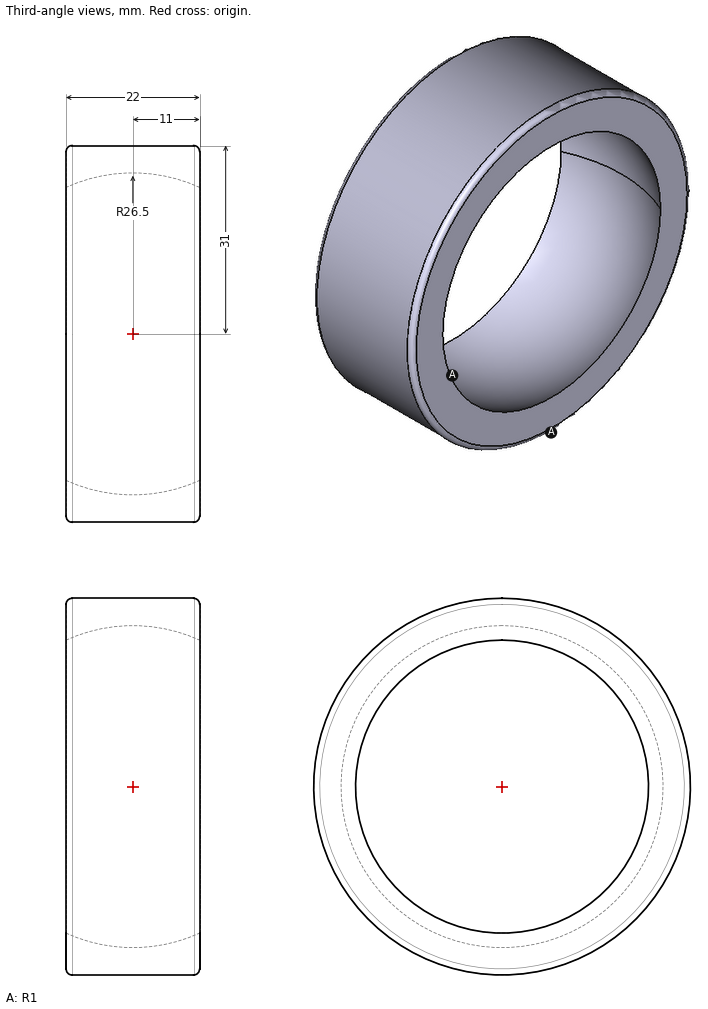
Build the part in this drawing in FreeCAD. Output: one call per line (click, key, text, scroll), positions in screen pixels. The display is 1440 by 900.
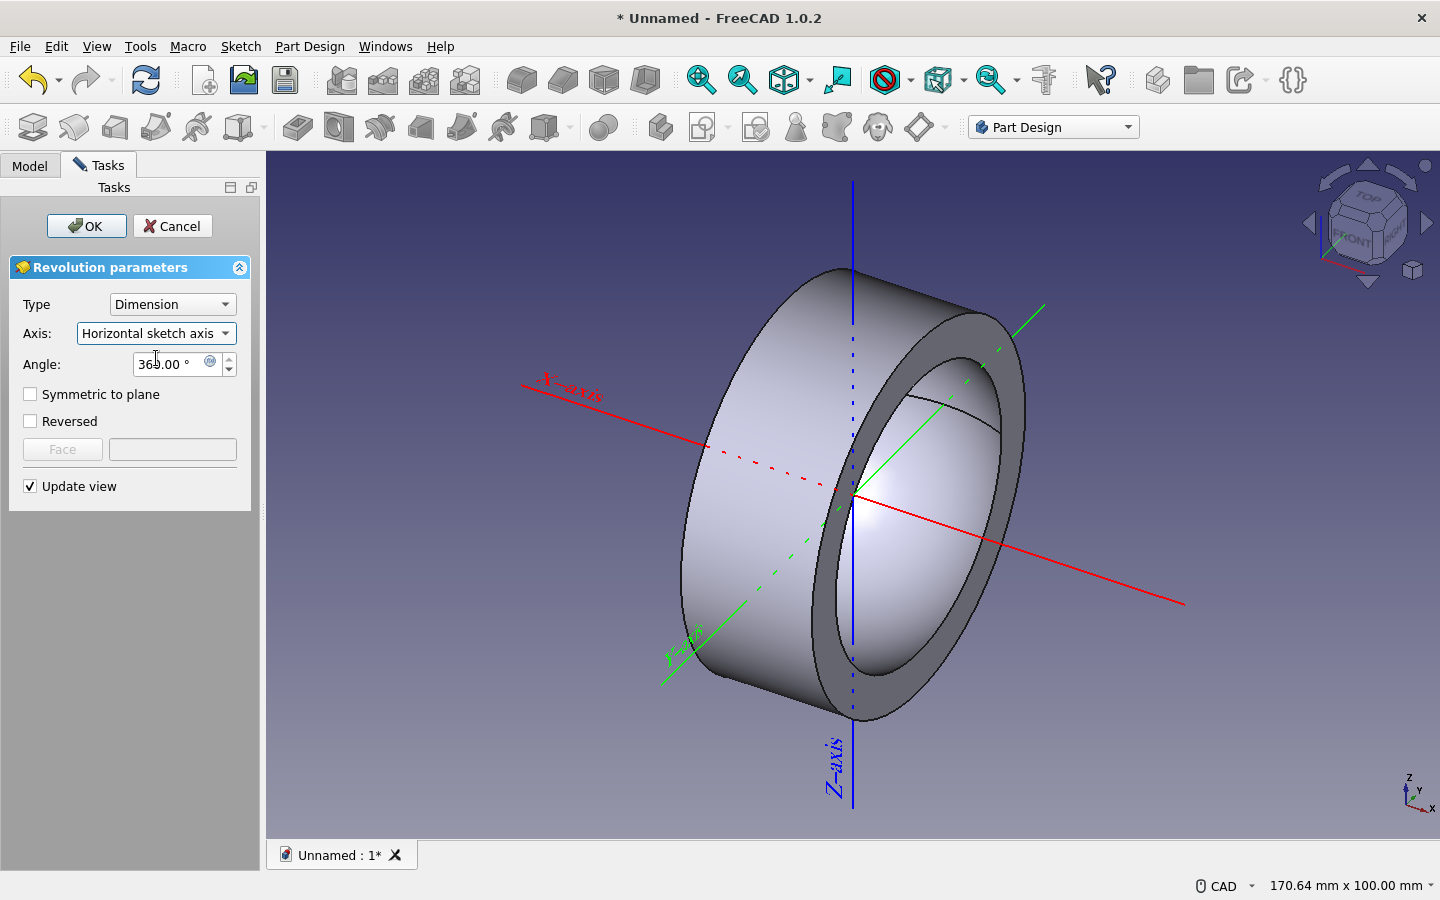
click(87, 226)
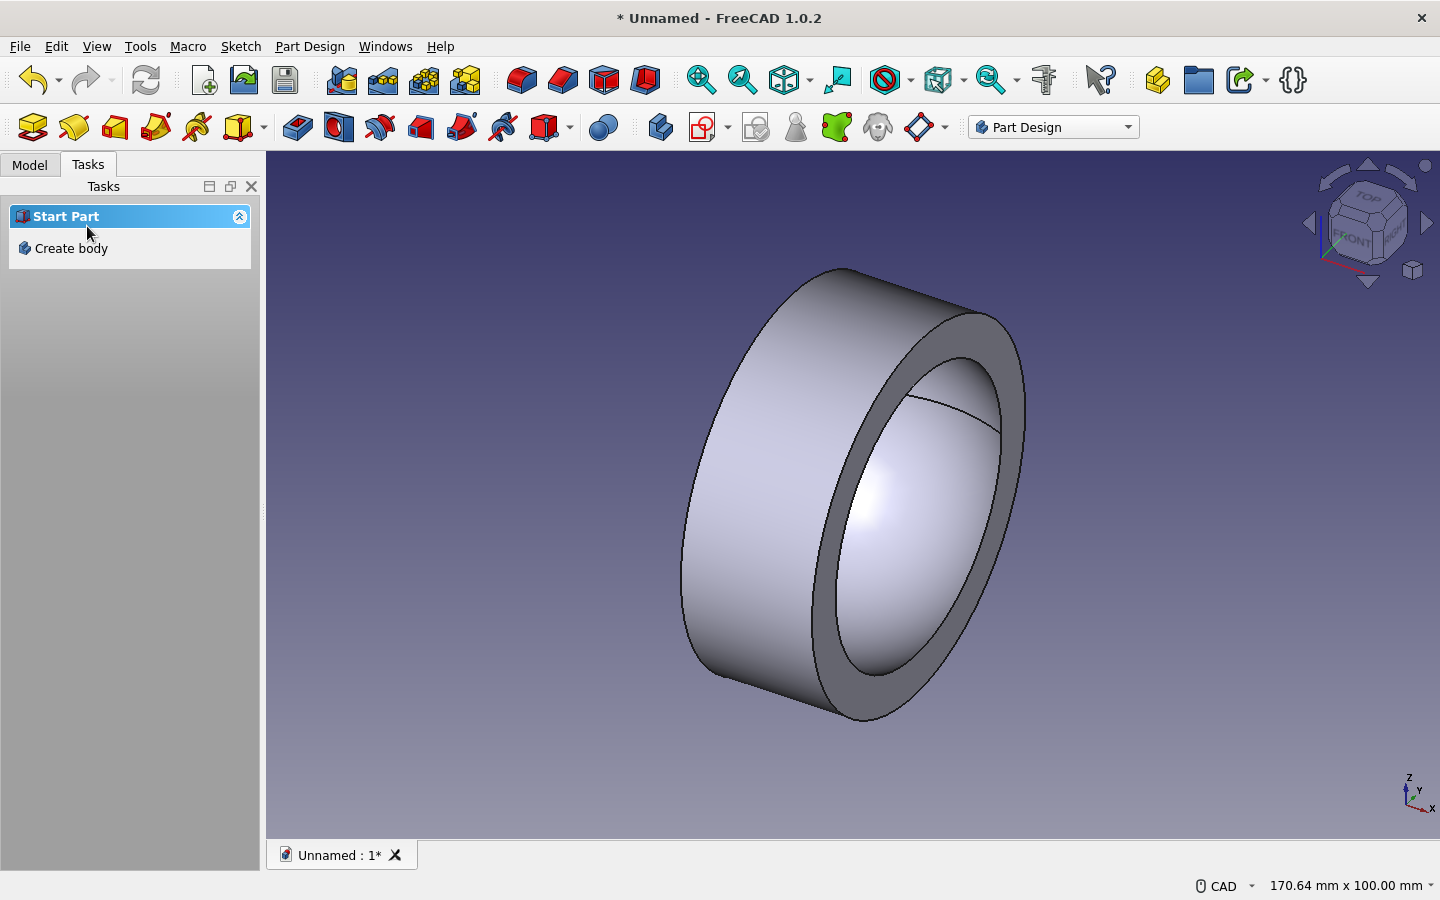
click(812, 622)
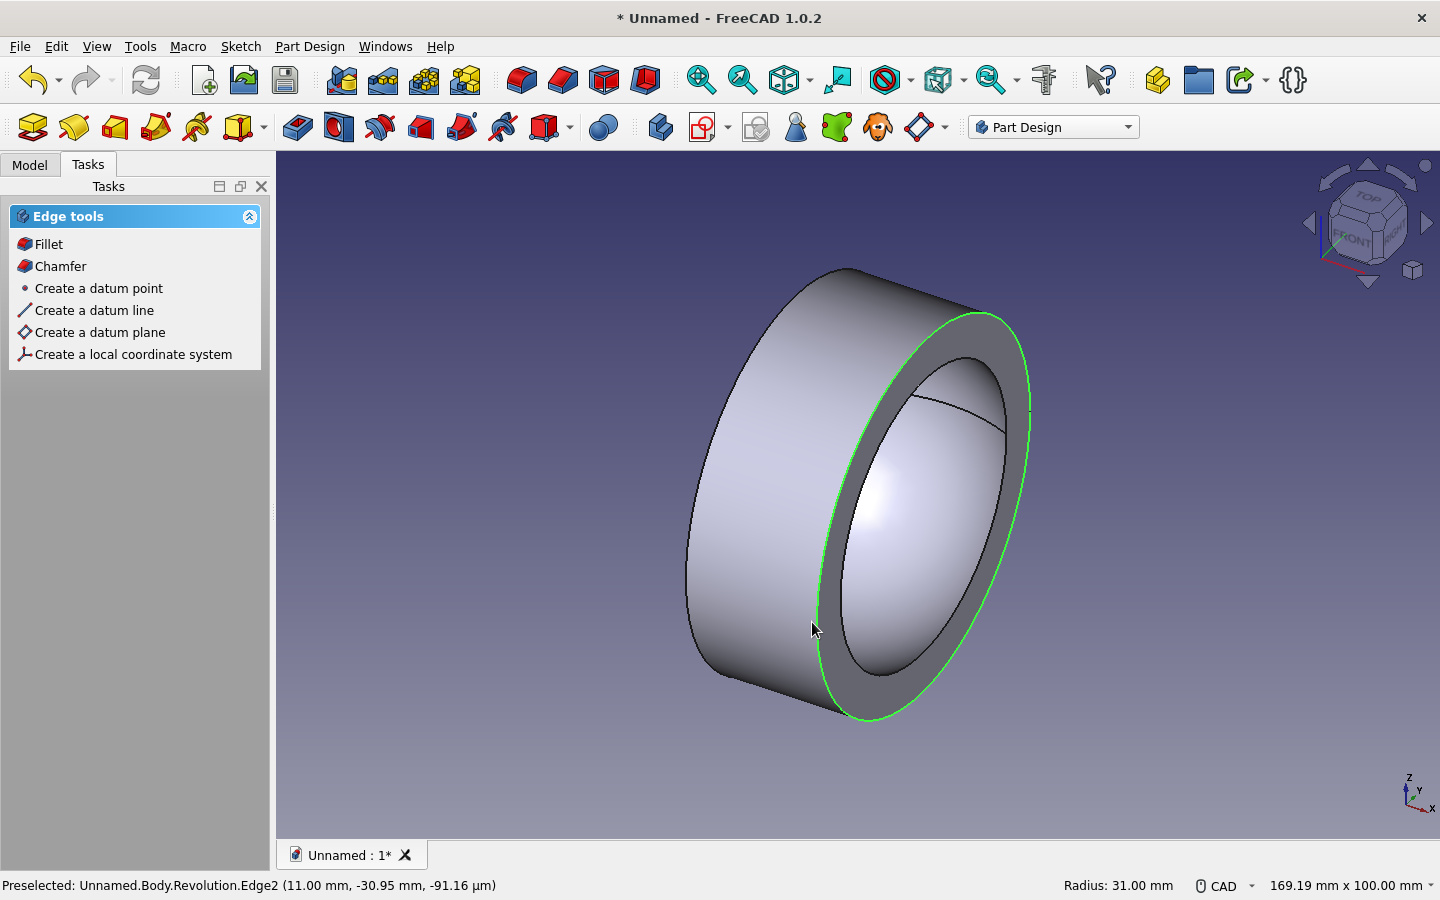
click(706, 661, ctrl)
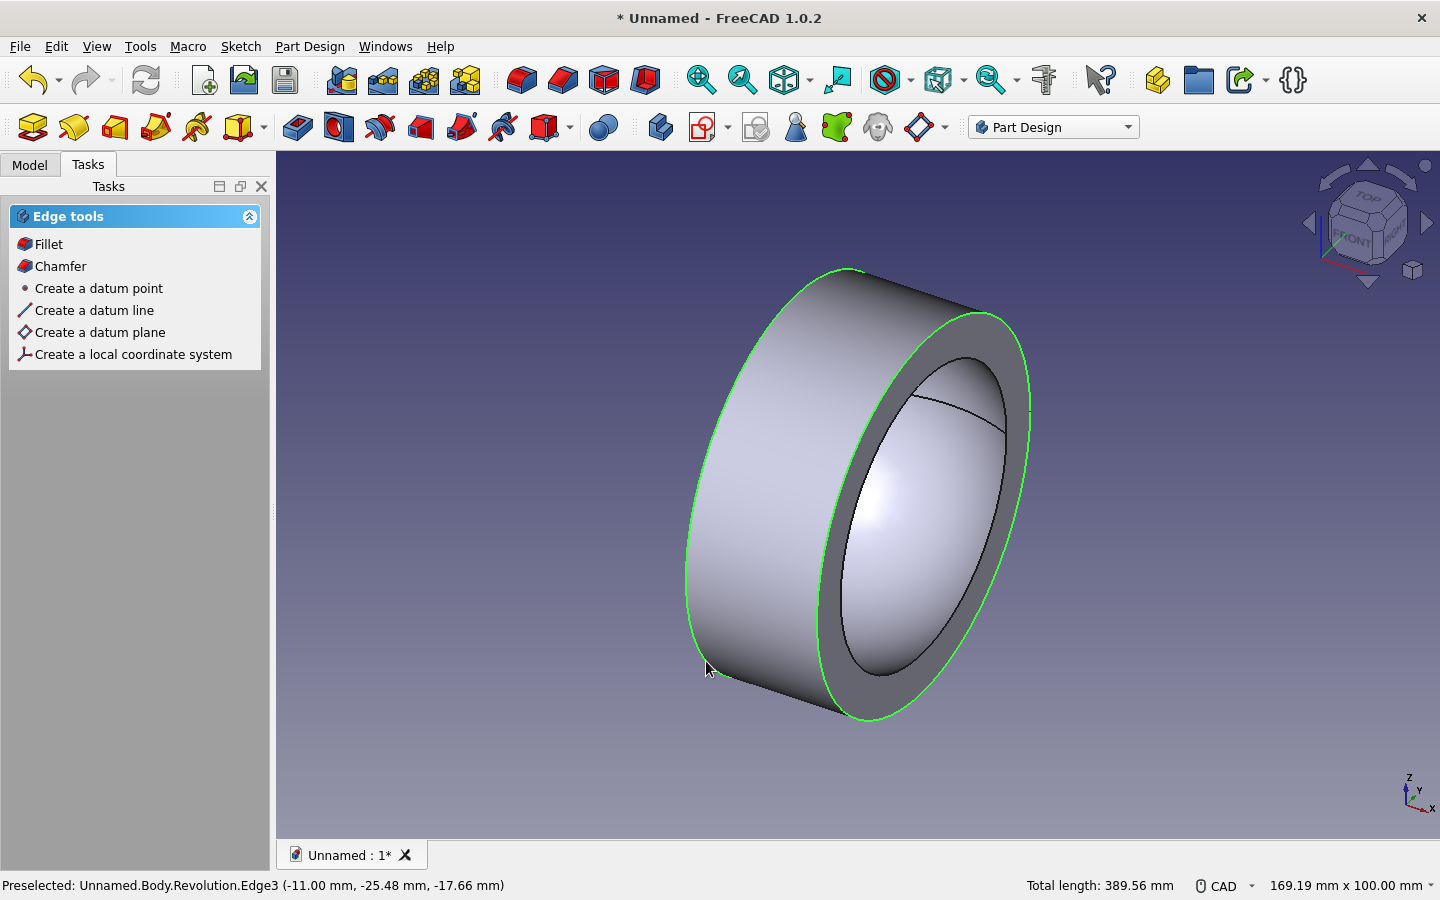
click(522, 80)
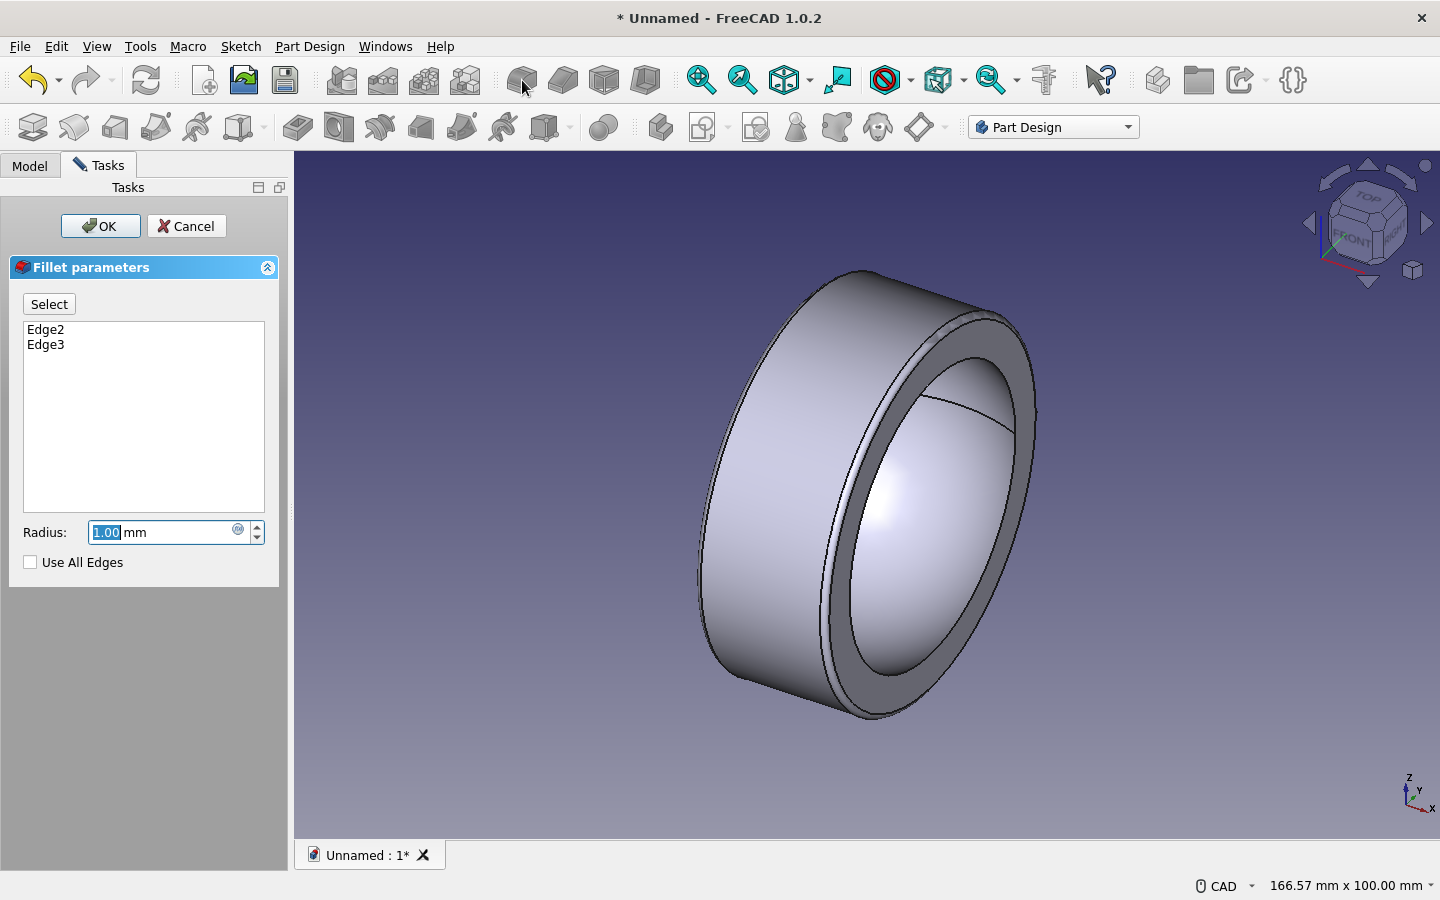
text(1)
key(Tab)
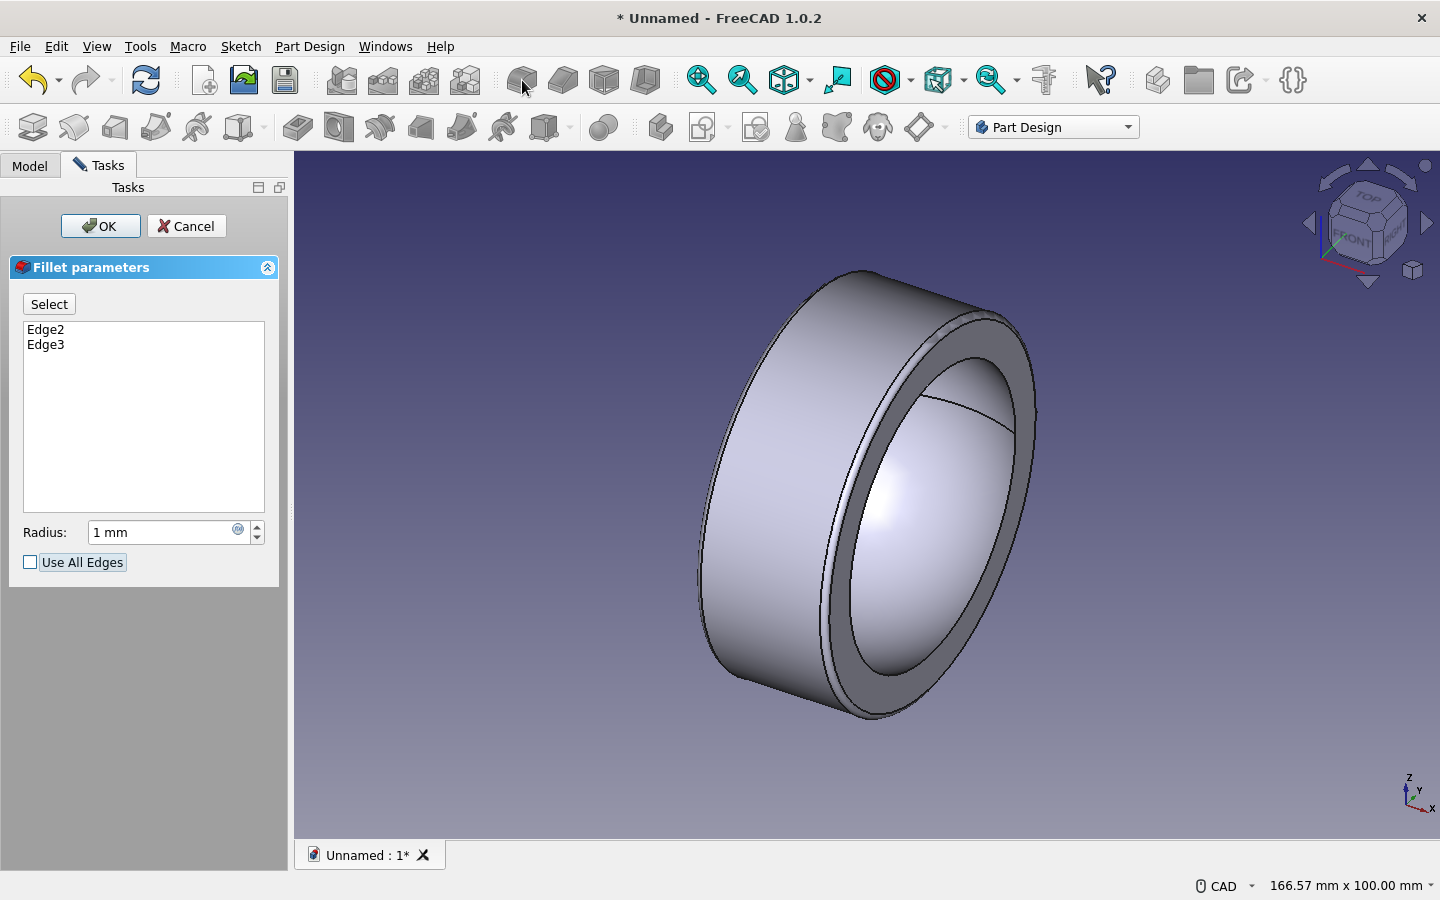
click(101, 226)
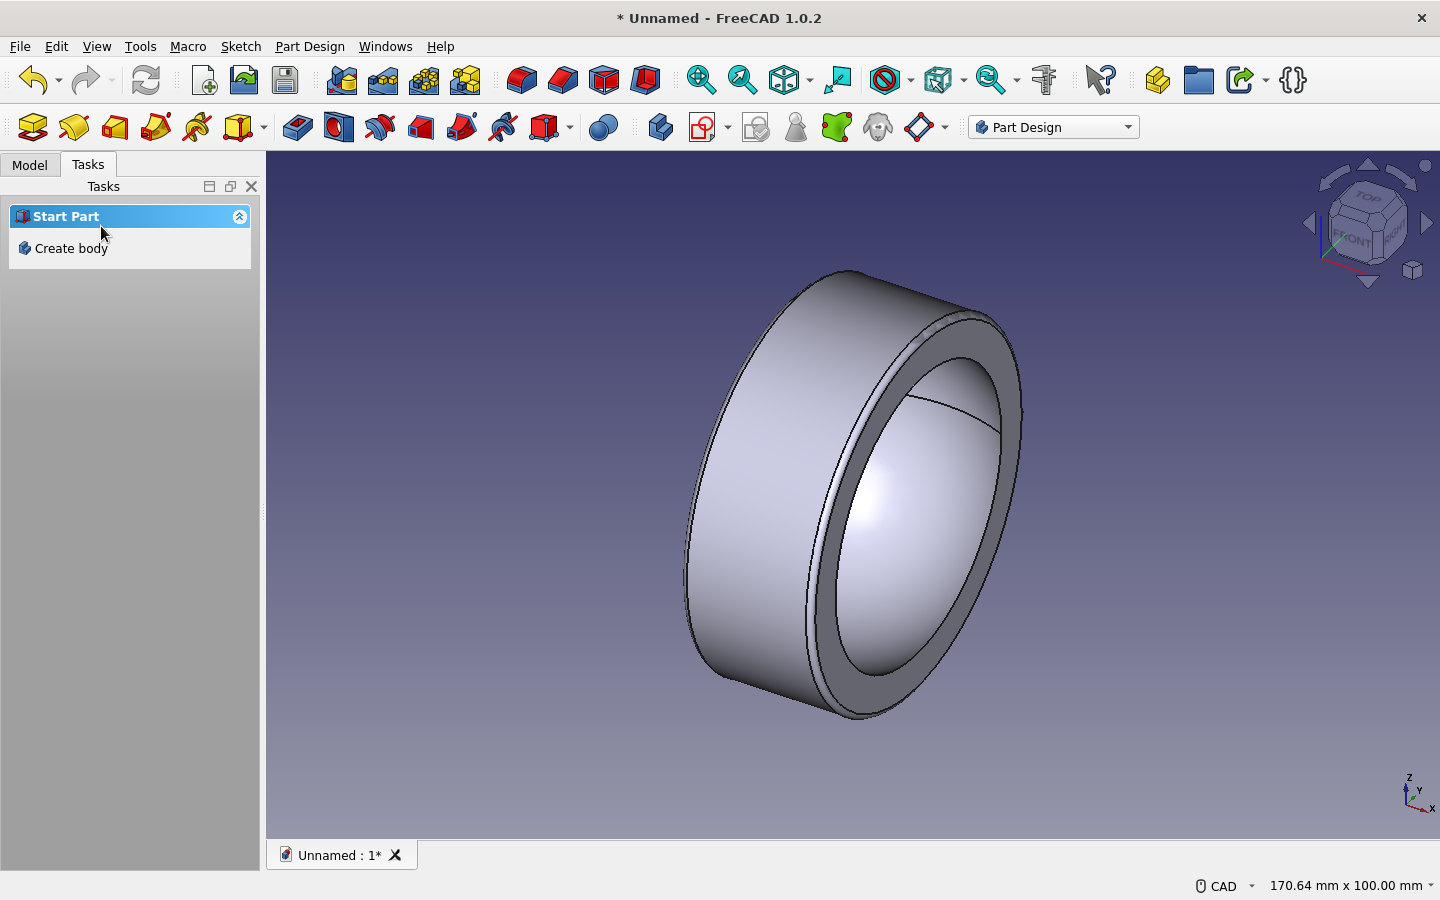
key(0)